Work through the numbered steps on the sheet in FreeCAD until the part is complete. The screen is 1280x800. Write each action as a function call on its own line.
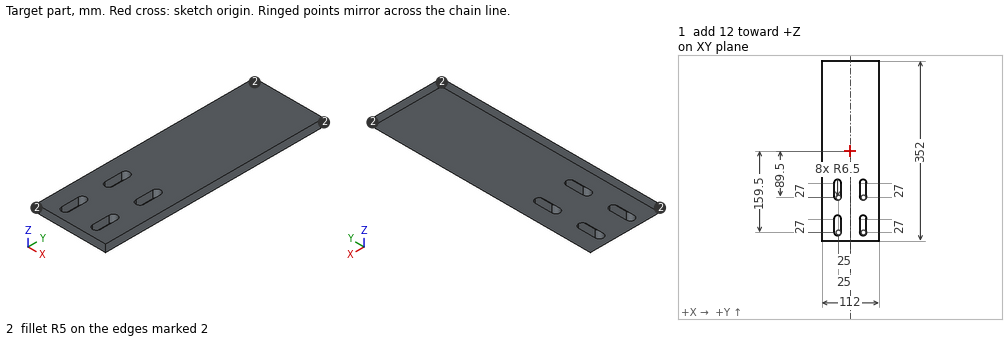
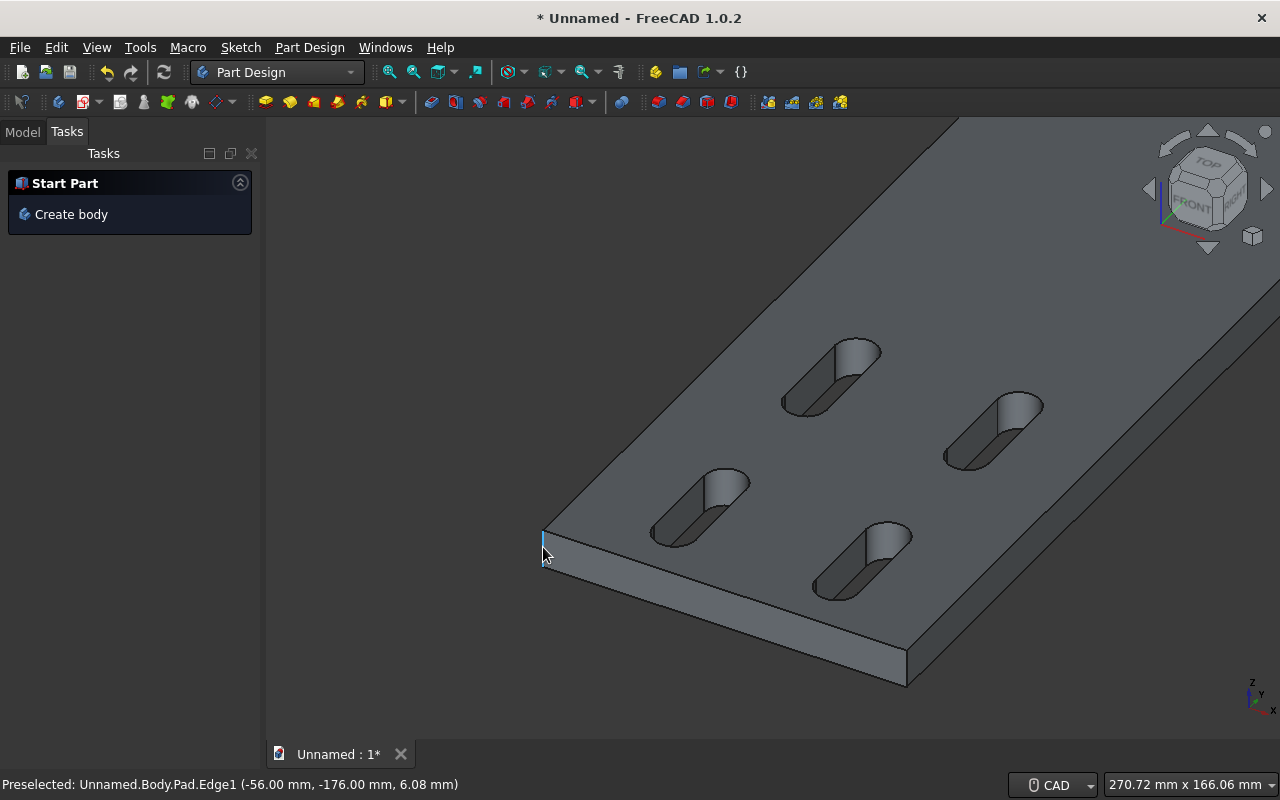
click(390, 72)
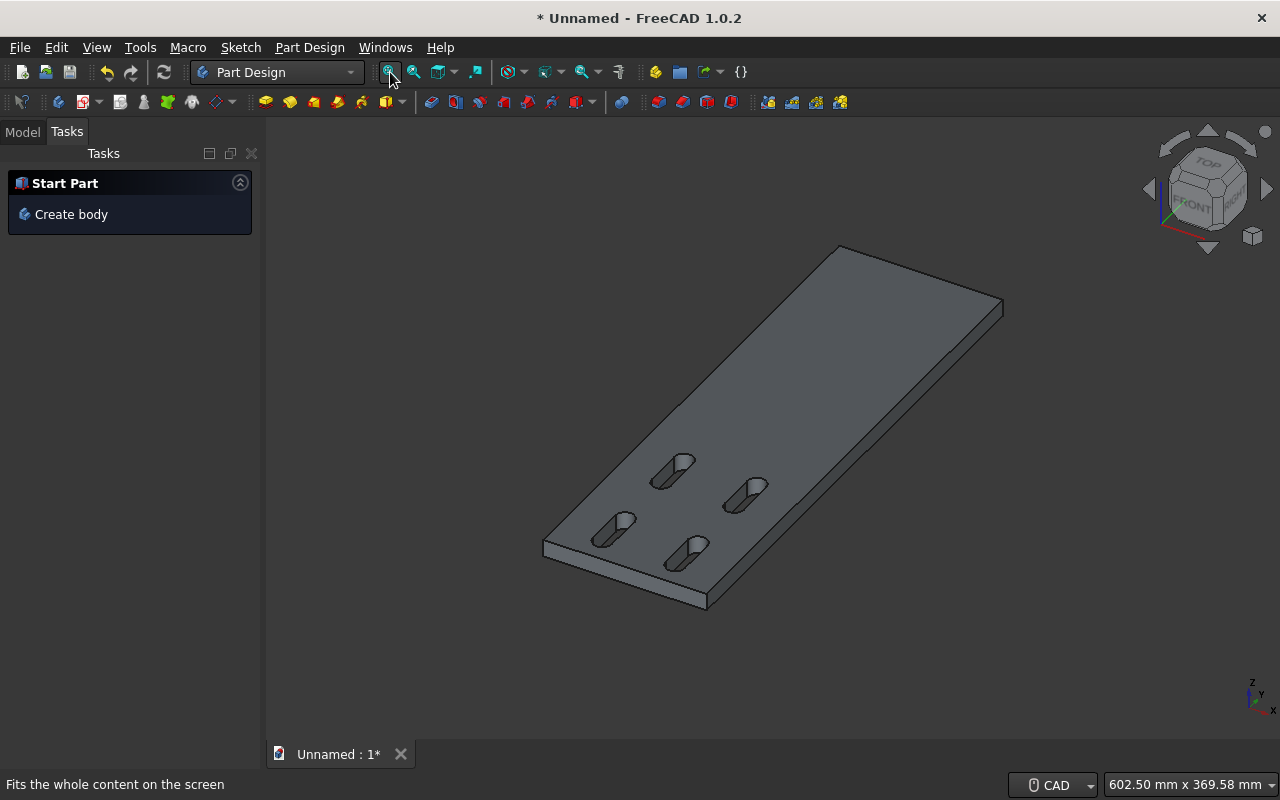
key(0)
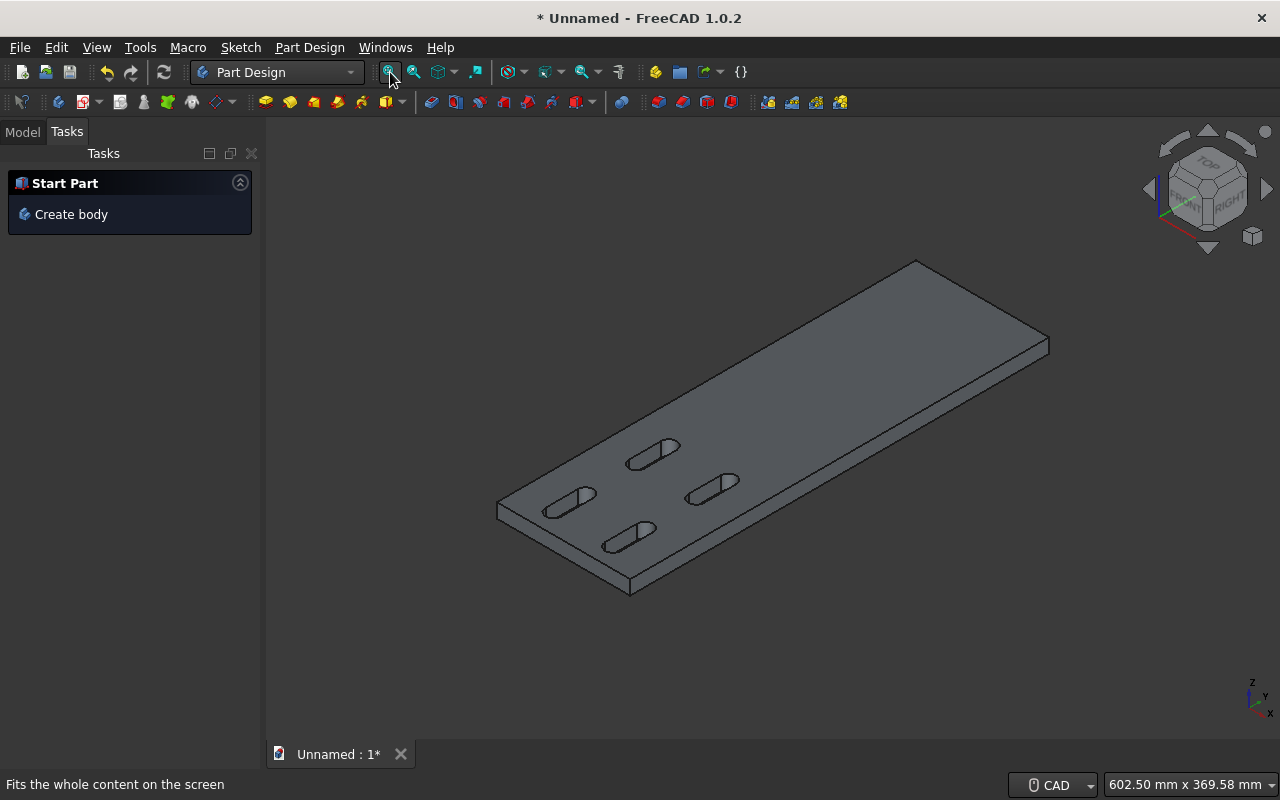
scroll(497, 509, up, 4)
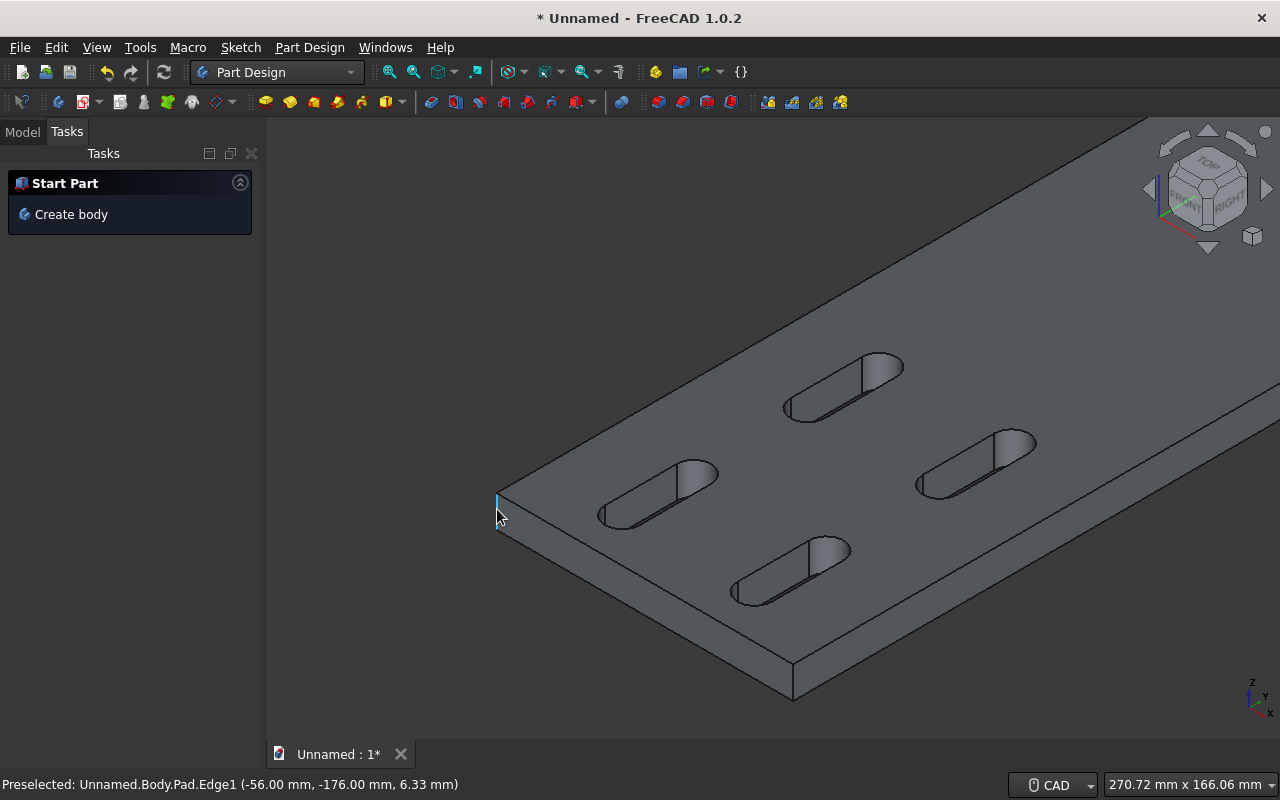
click(390, 72)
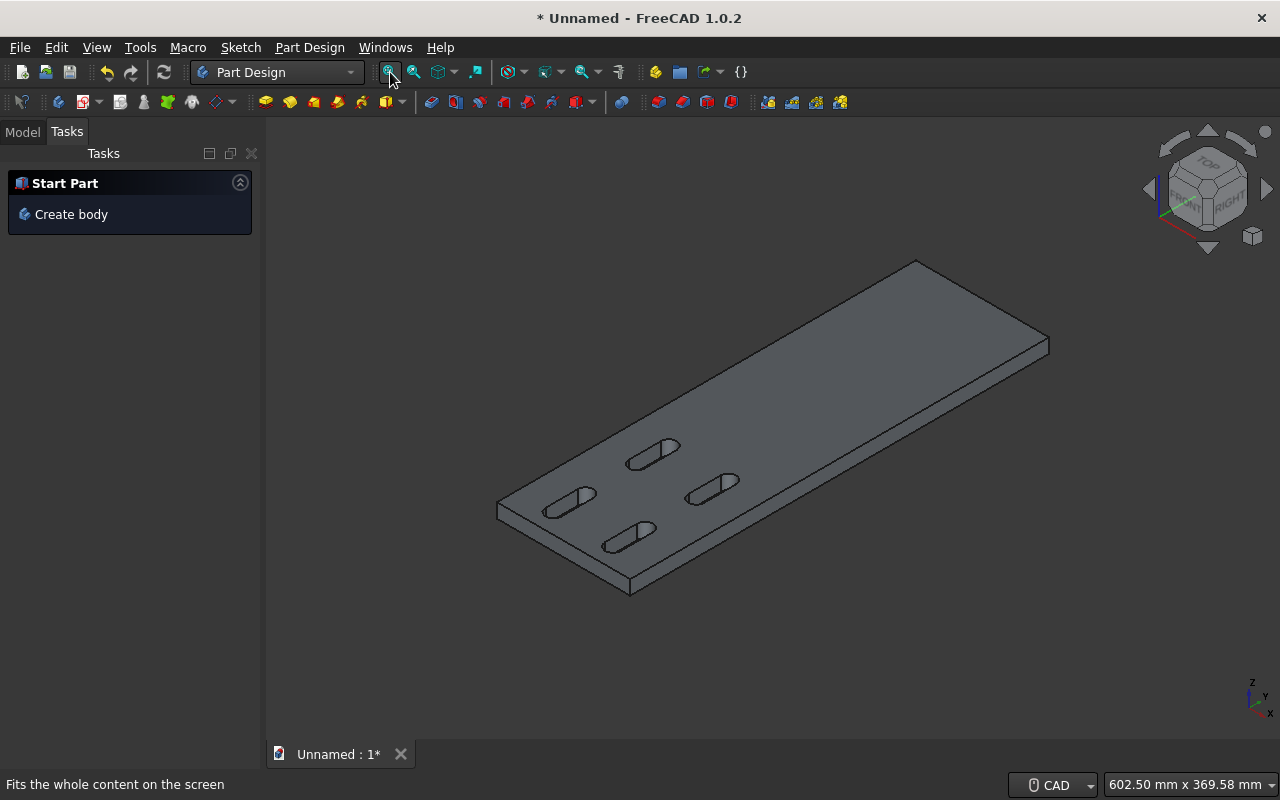
key(2)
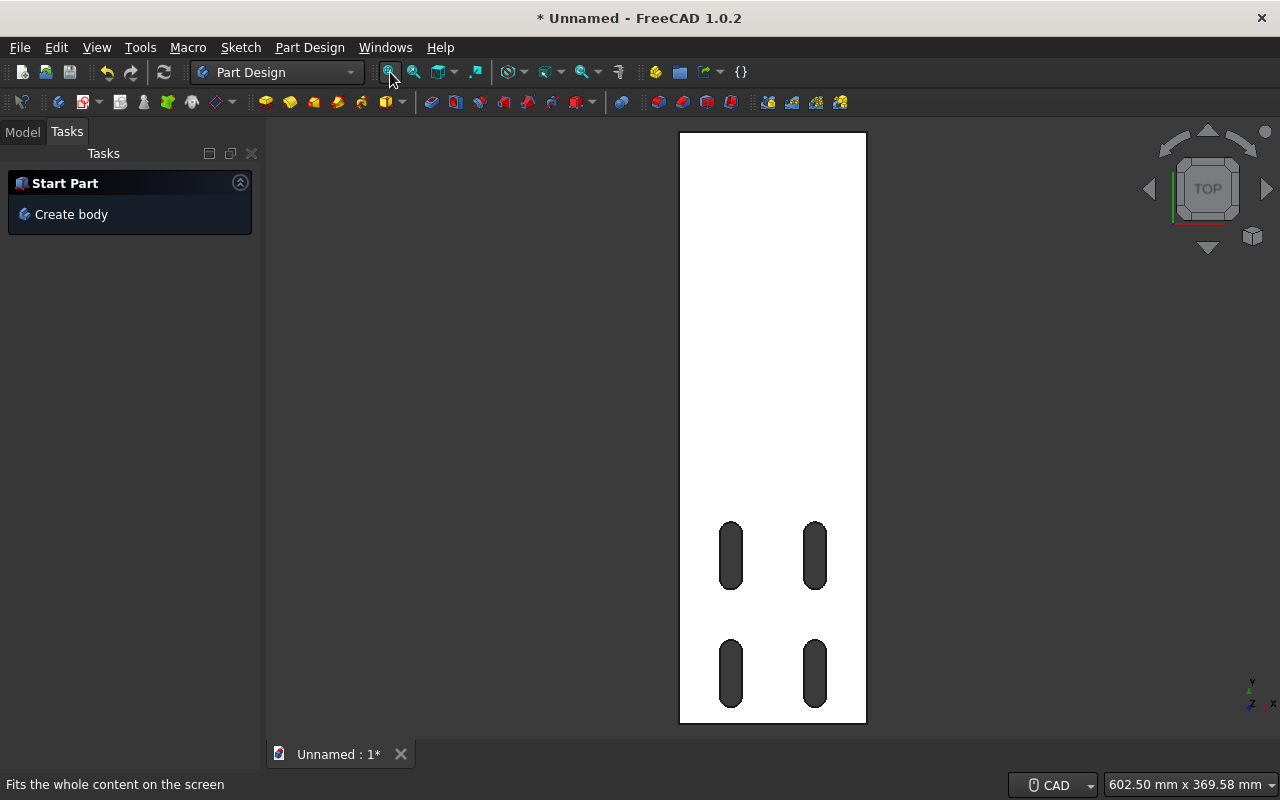
key(1)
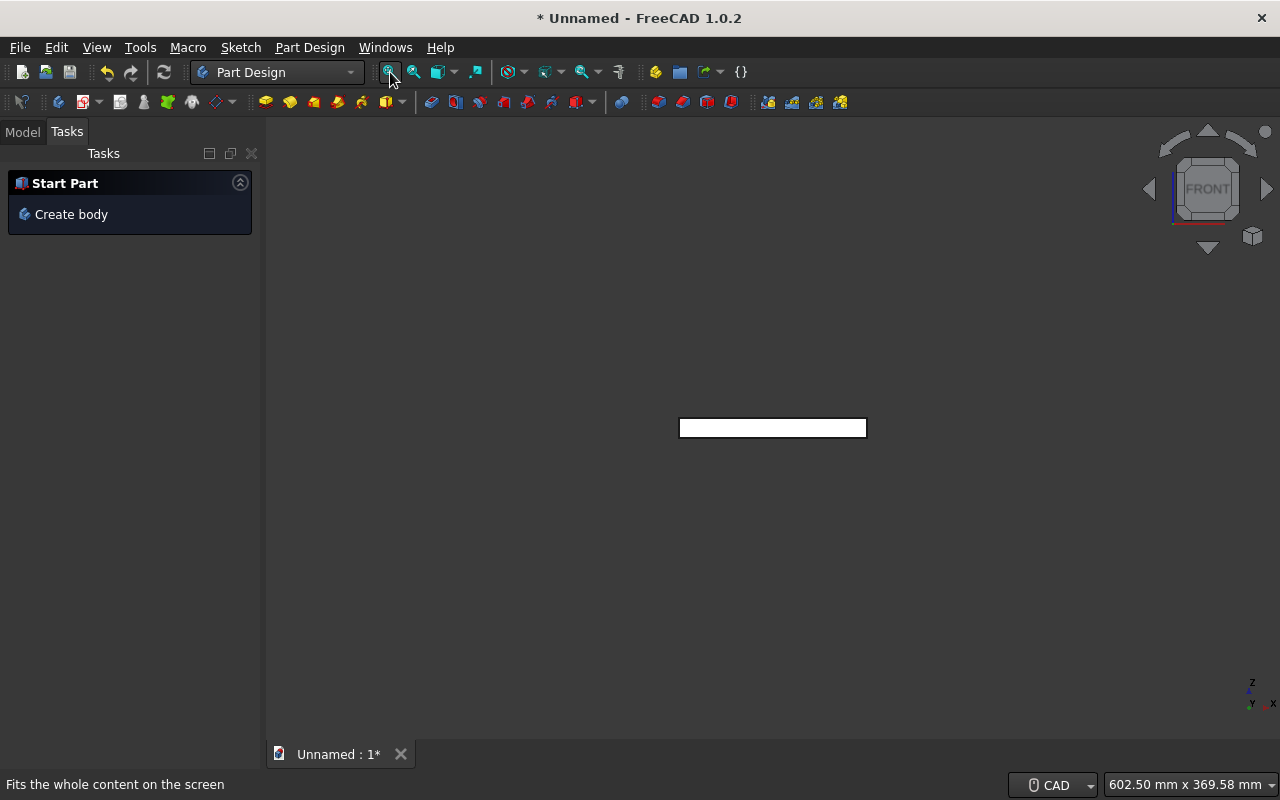
click(390, 72)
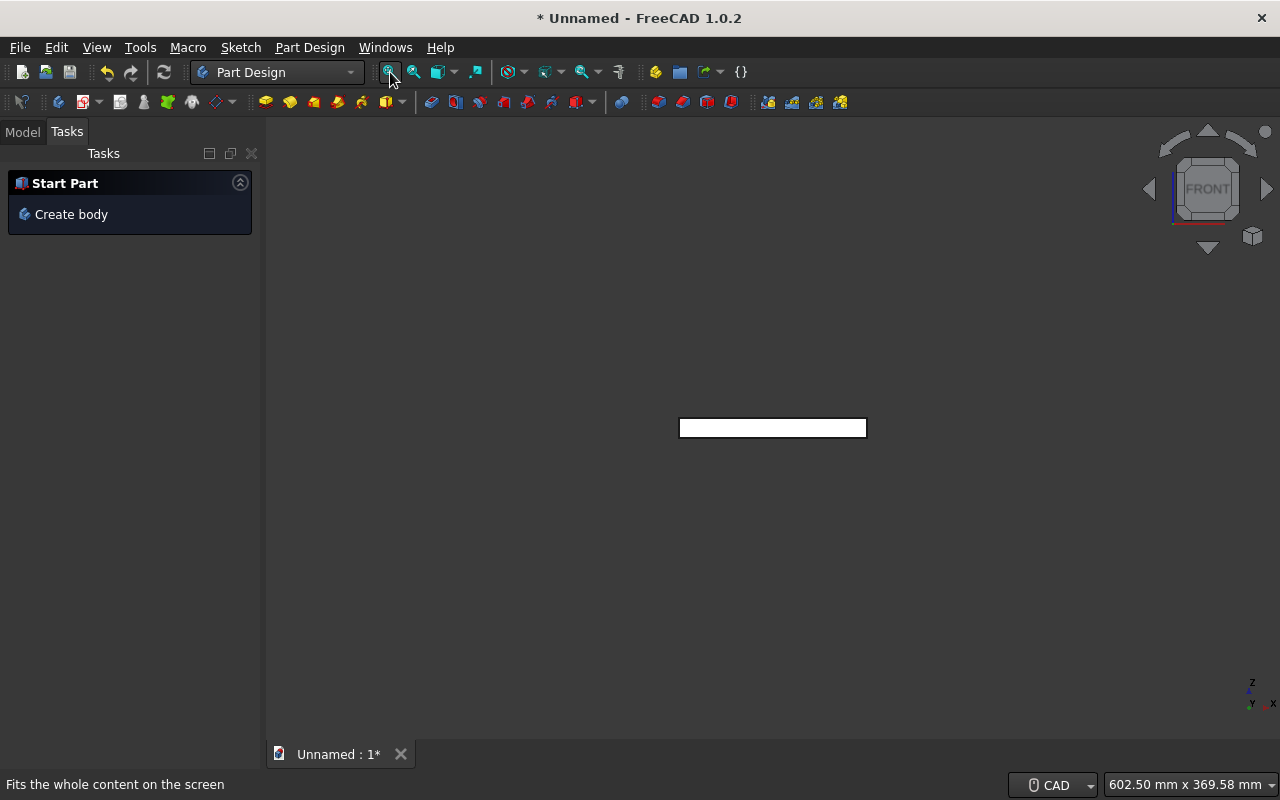
click(679, 427)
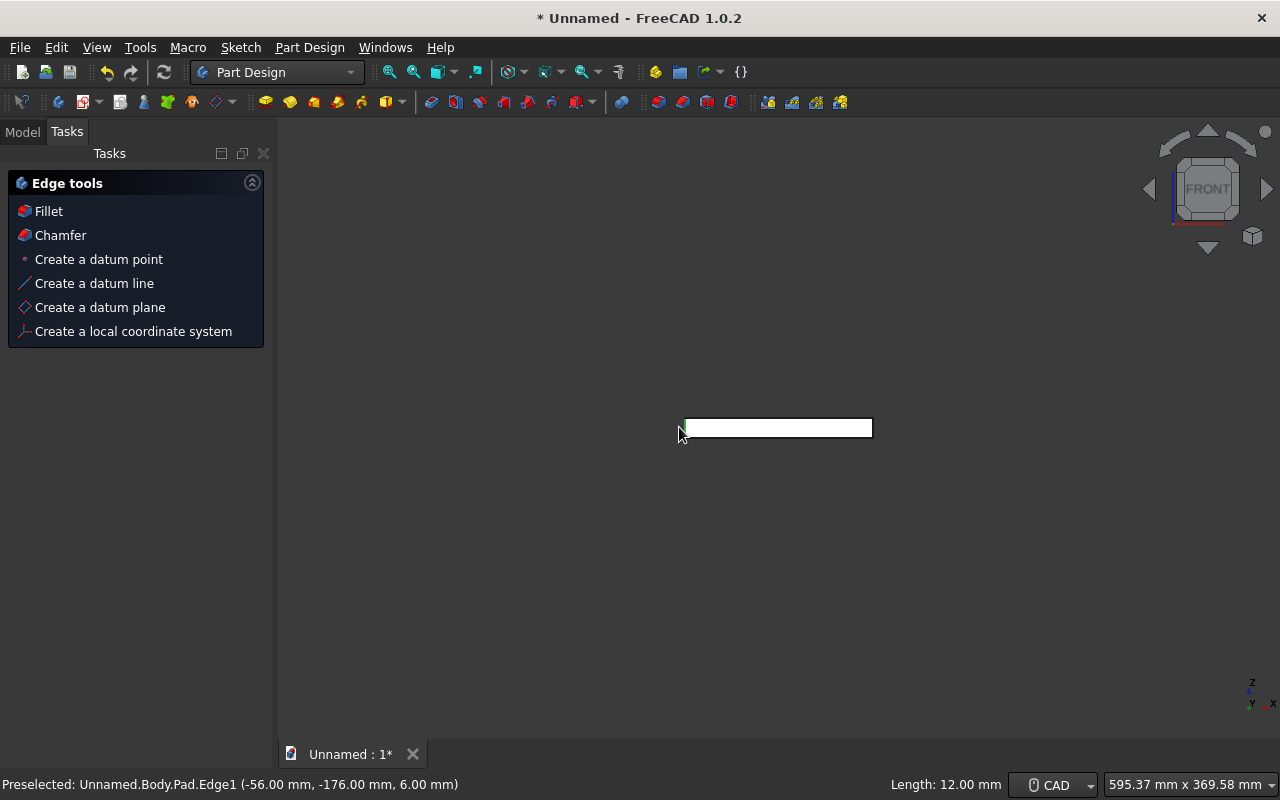
scroll(685, 427, up, 4)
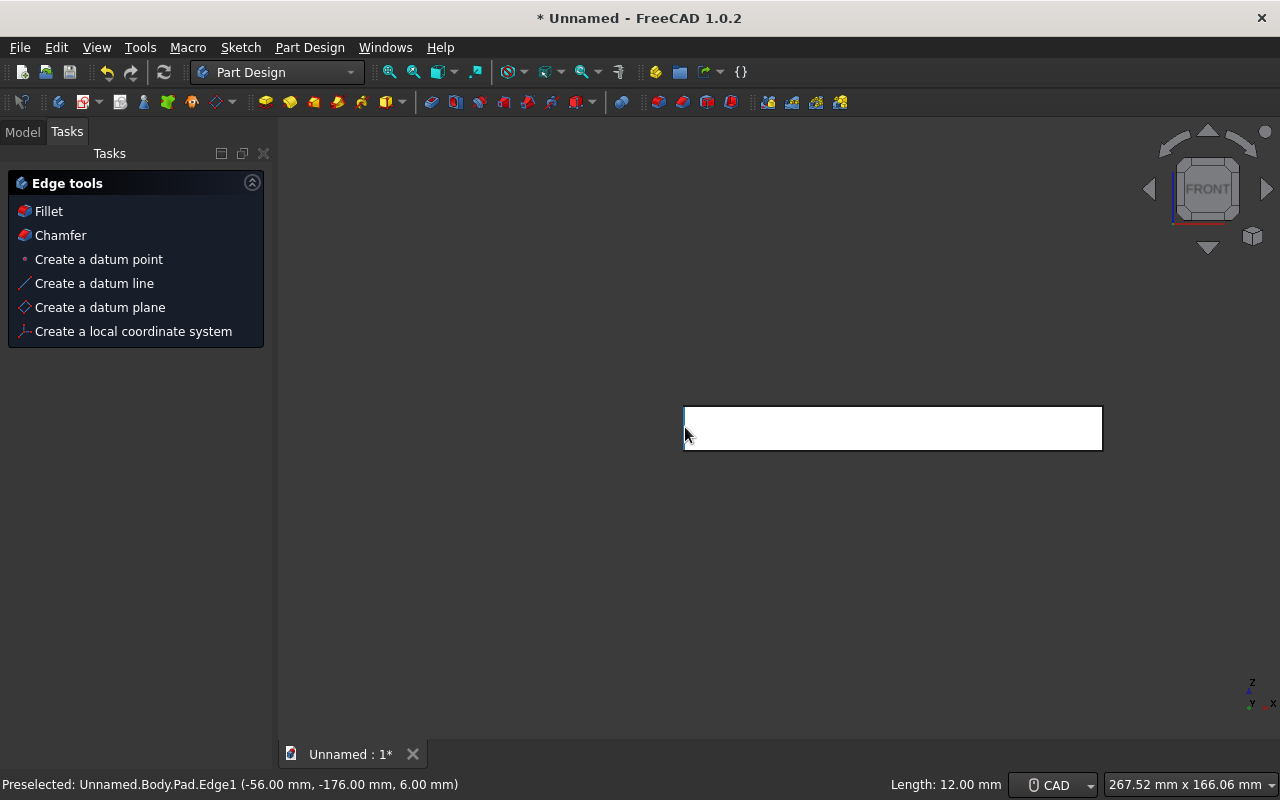
click(390, 72)